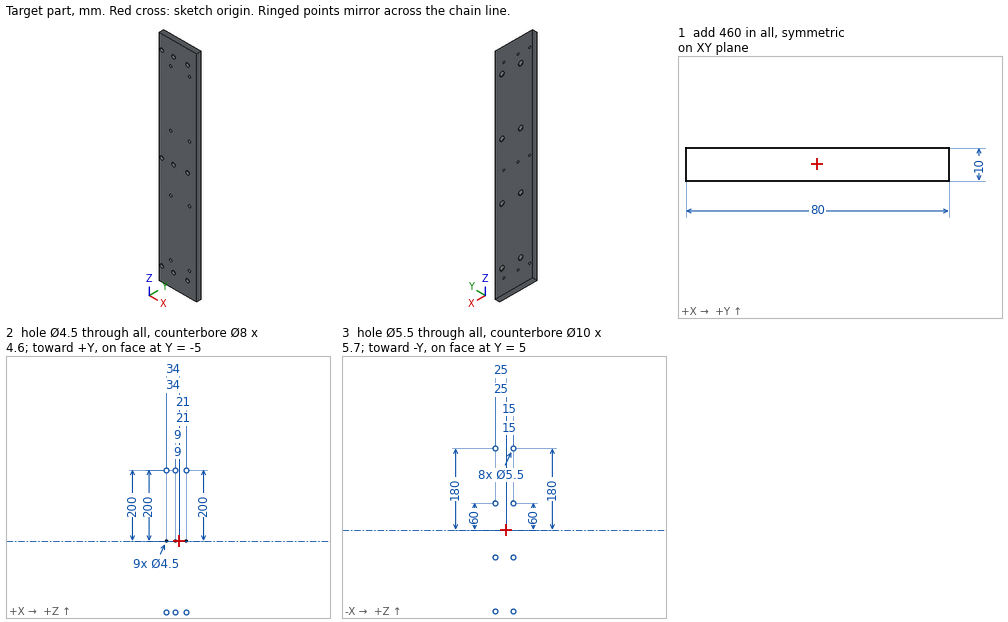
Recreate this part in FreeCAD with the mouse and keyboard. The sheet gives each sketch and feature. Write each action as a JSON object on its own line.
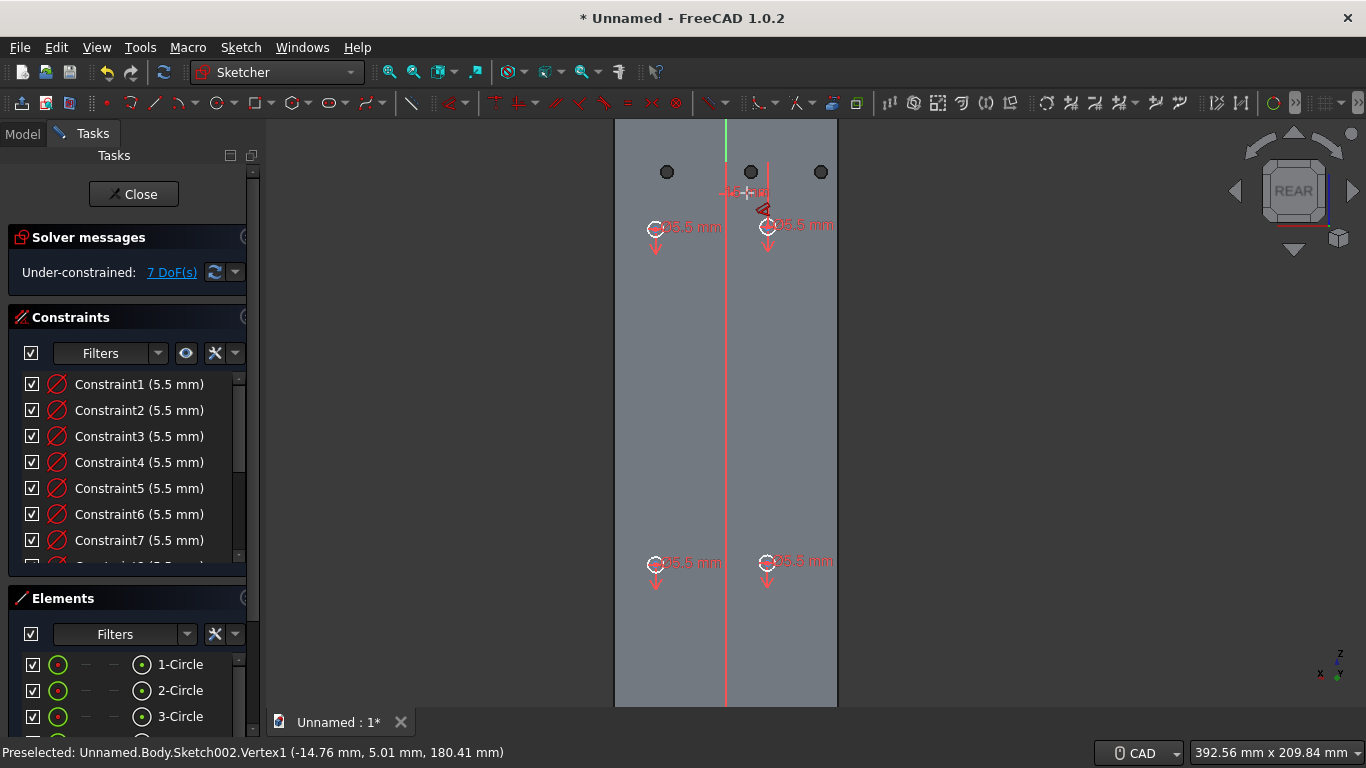
{"action": "left_click", "coordinate": [656, 229]}
{"action": "left_click", "coordinate": [675, 195]}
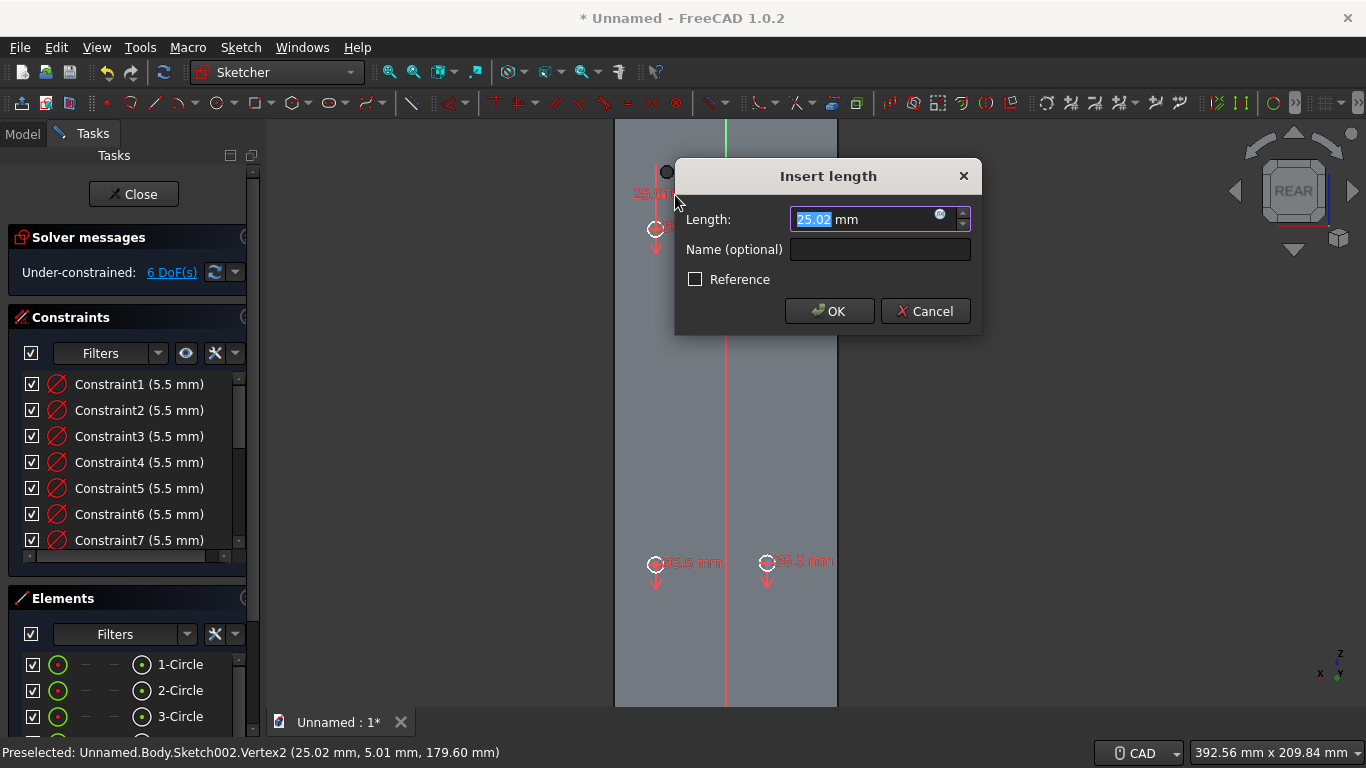
{"action": "type", "text": "25"}
{"action": "key", "text": "Return"}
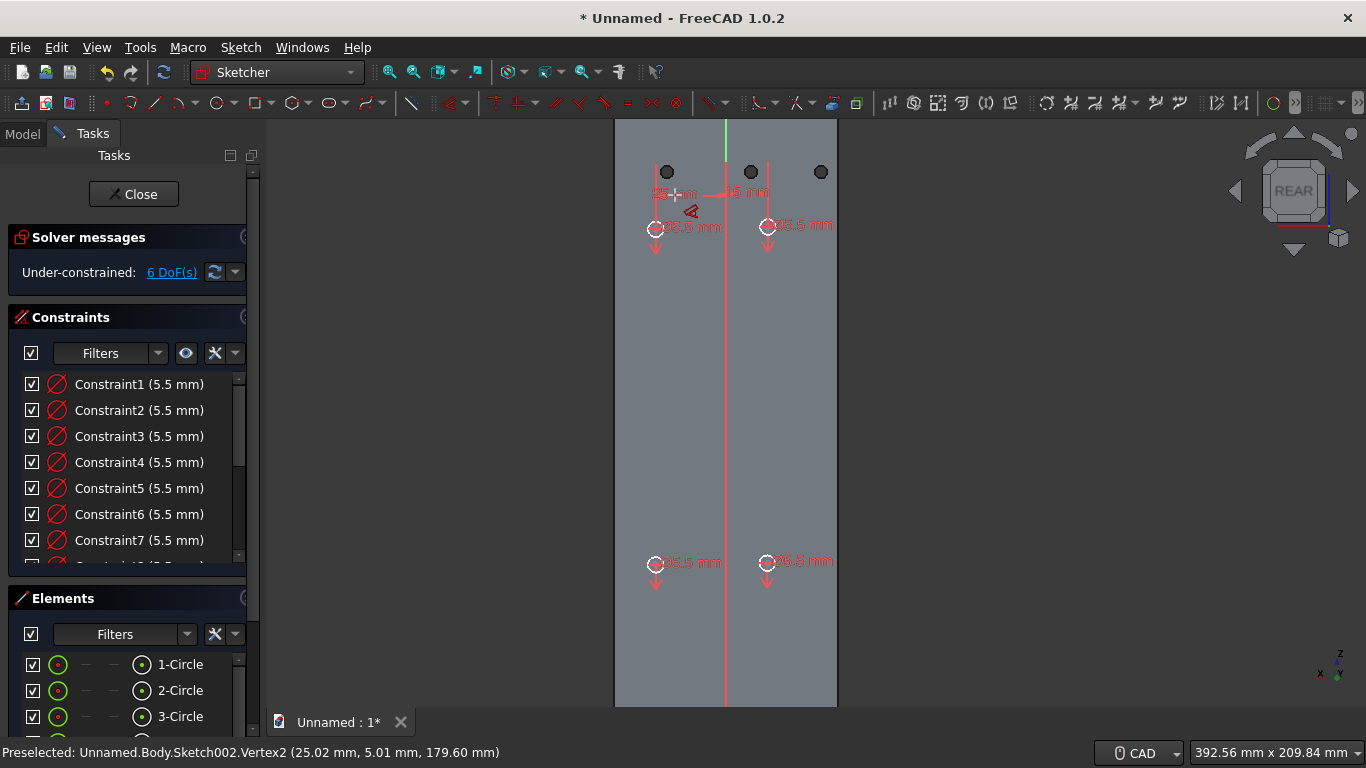
{"action": "left_click", "coordinate": [767, 563]}
{"action": "left_click", "coordinate": [747, 529]}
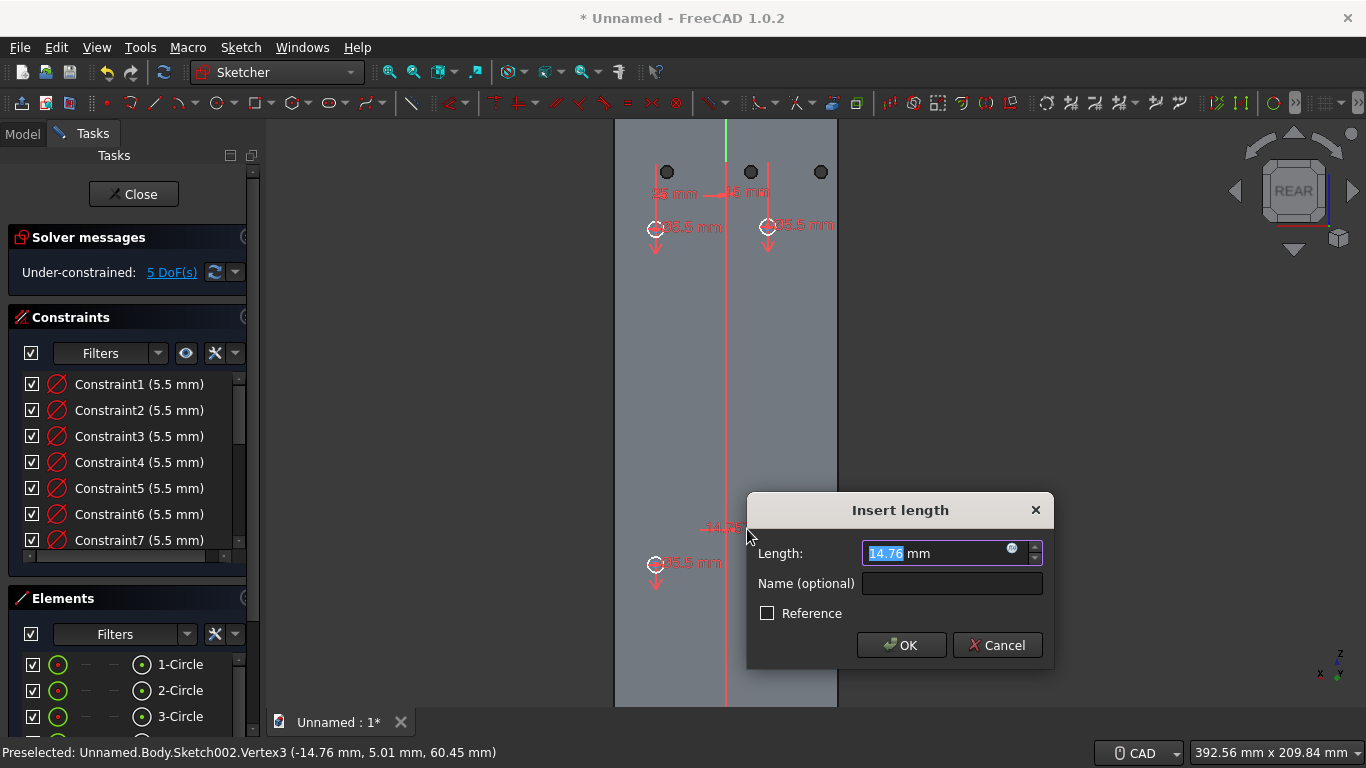
{"action": "type", "text": "15"}
{"action": "key", "text": "Return"}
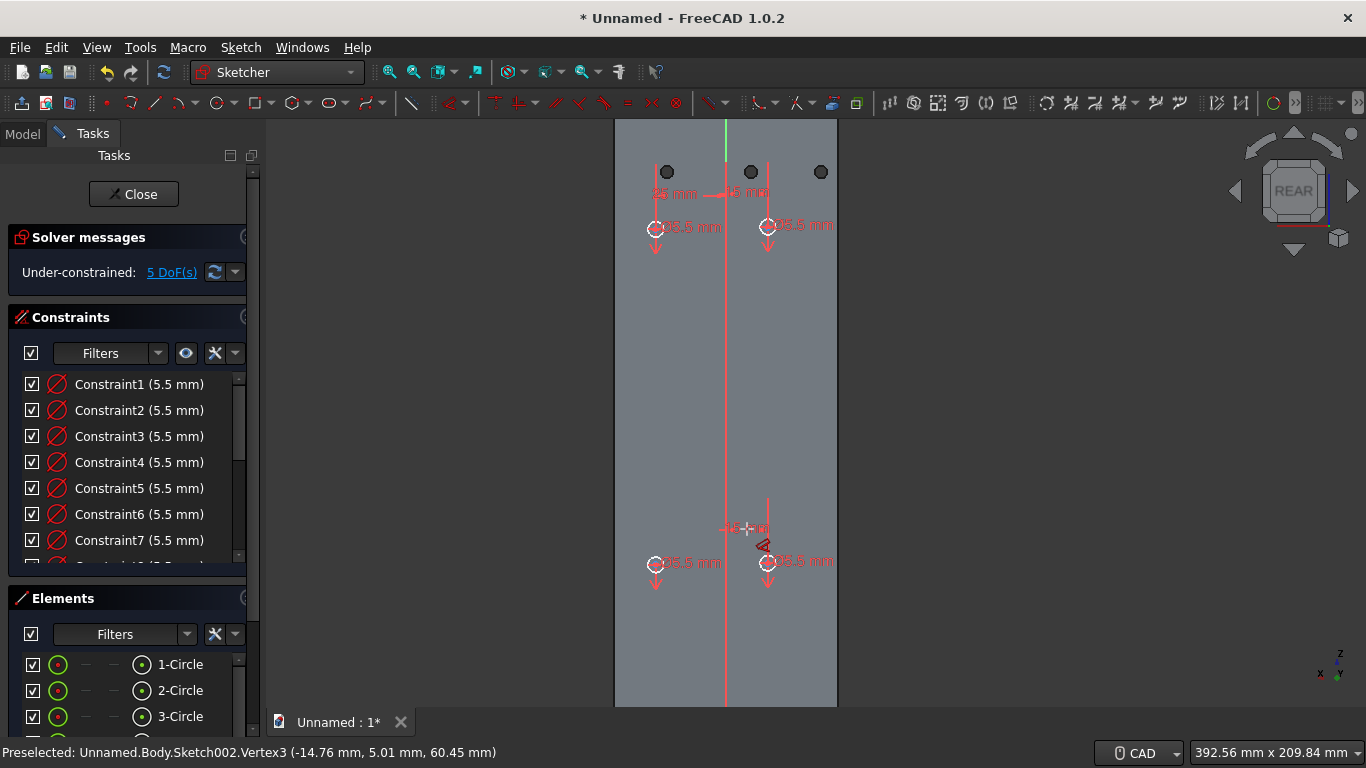
{"action": "left_click", "coordinate": [768, 563]}
{"action": "left_click", "coordinate": [802, 621]}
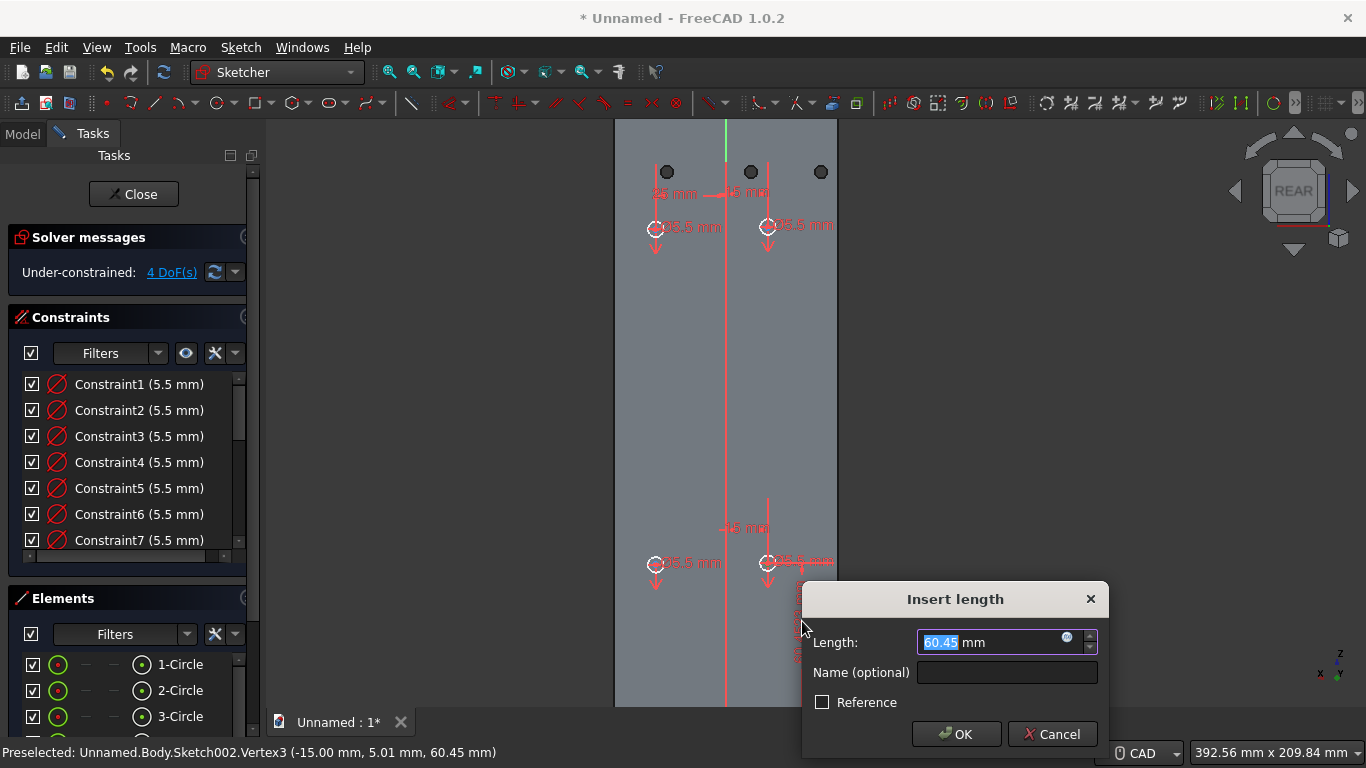
{"action": "type", "text": "60"}
{"action": "key", "text": "Return"}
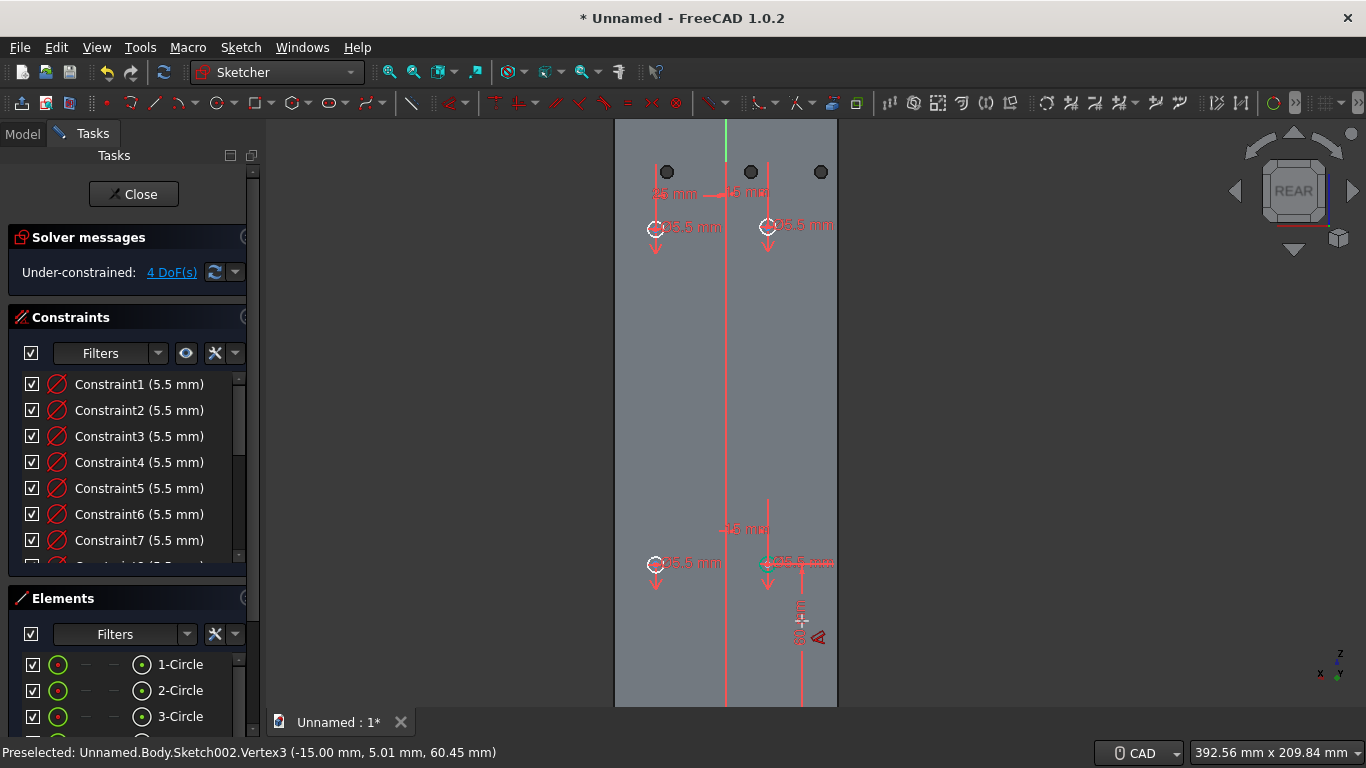
{"action": "left_click", "coordinate": [656, 565]}
{"action": "left_click", "coordinate": [675, 531]}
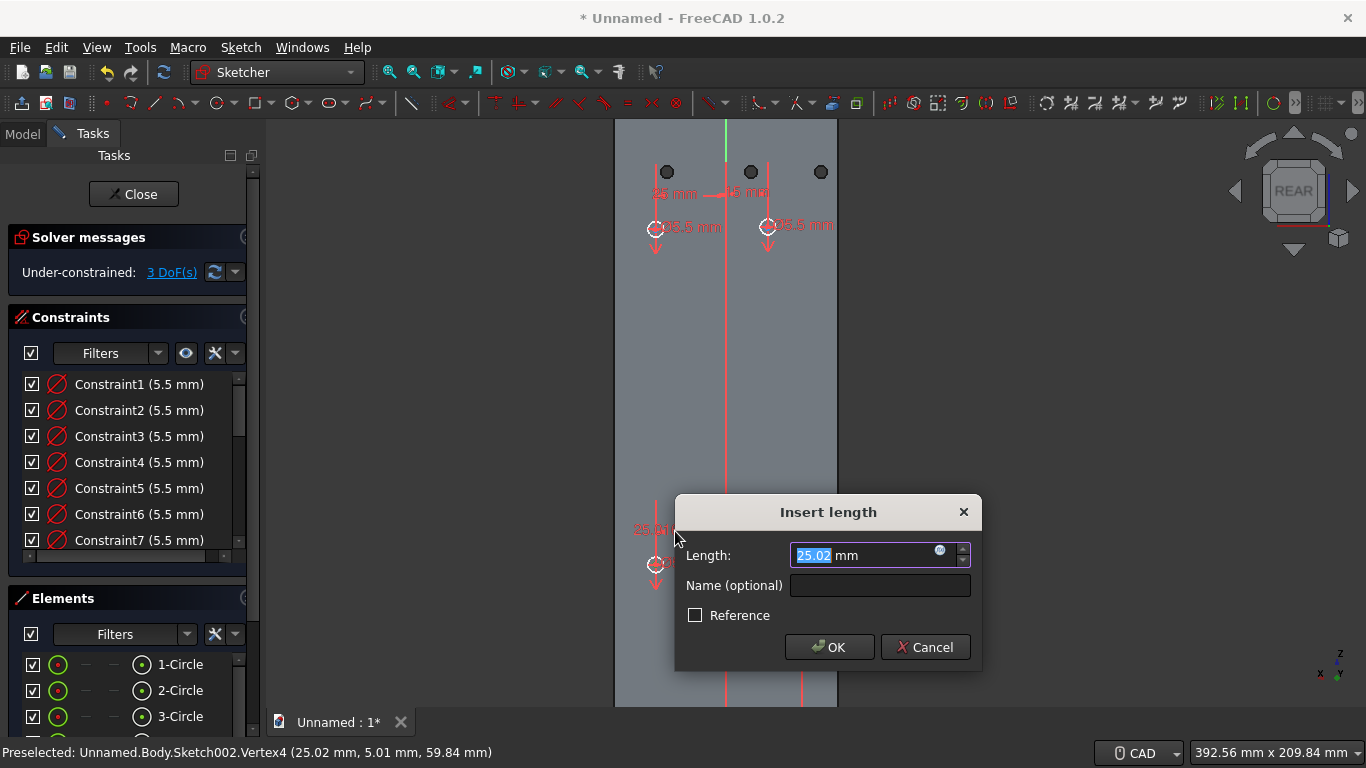
{"action": "type", "text": "25"}
{"action": "key", "text": "Return"}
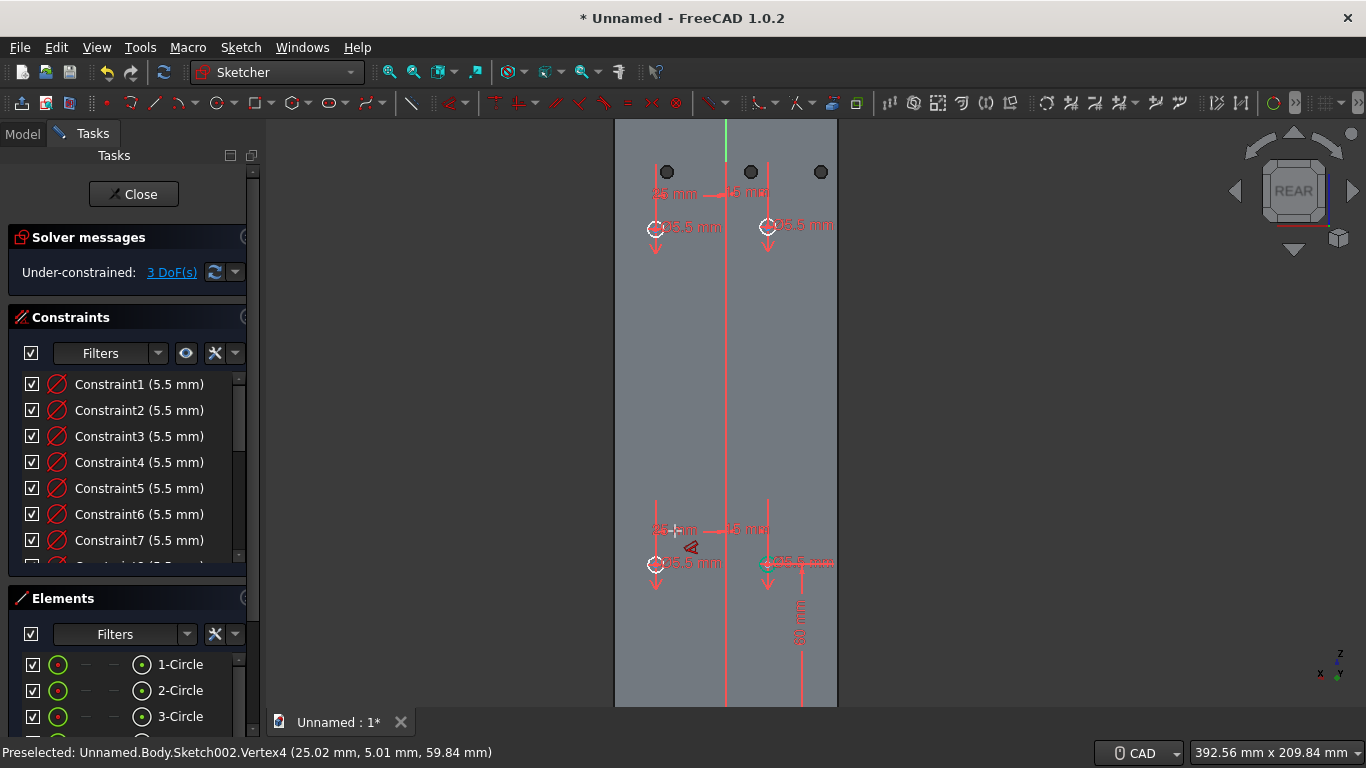
{"action": "left_click", "coordinate": [656, 565]}
{"action": "left_click", "coordinate": [622, 622]}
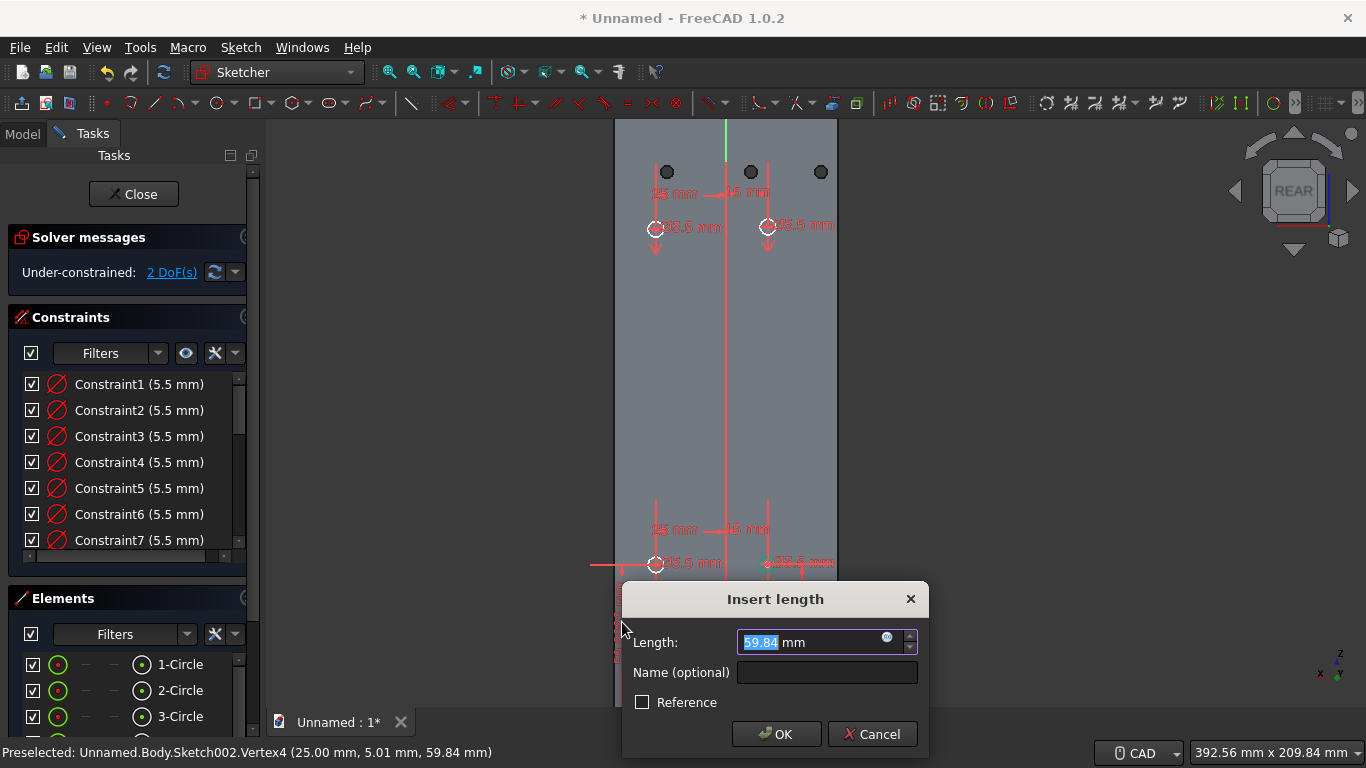
{"action": "type", "text": "60"}
{"action": "key", "text": "Return"}